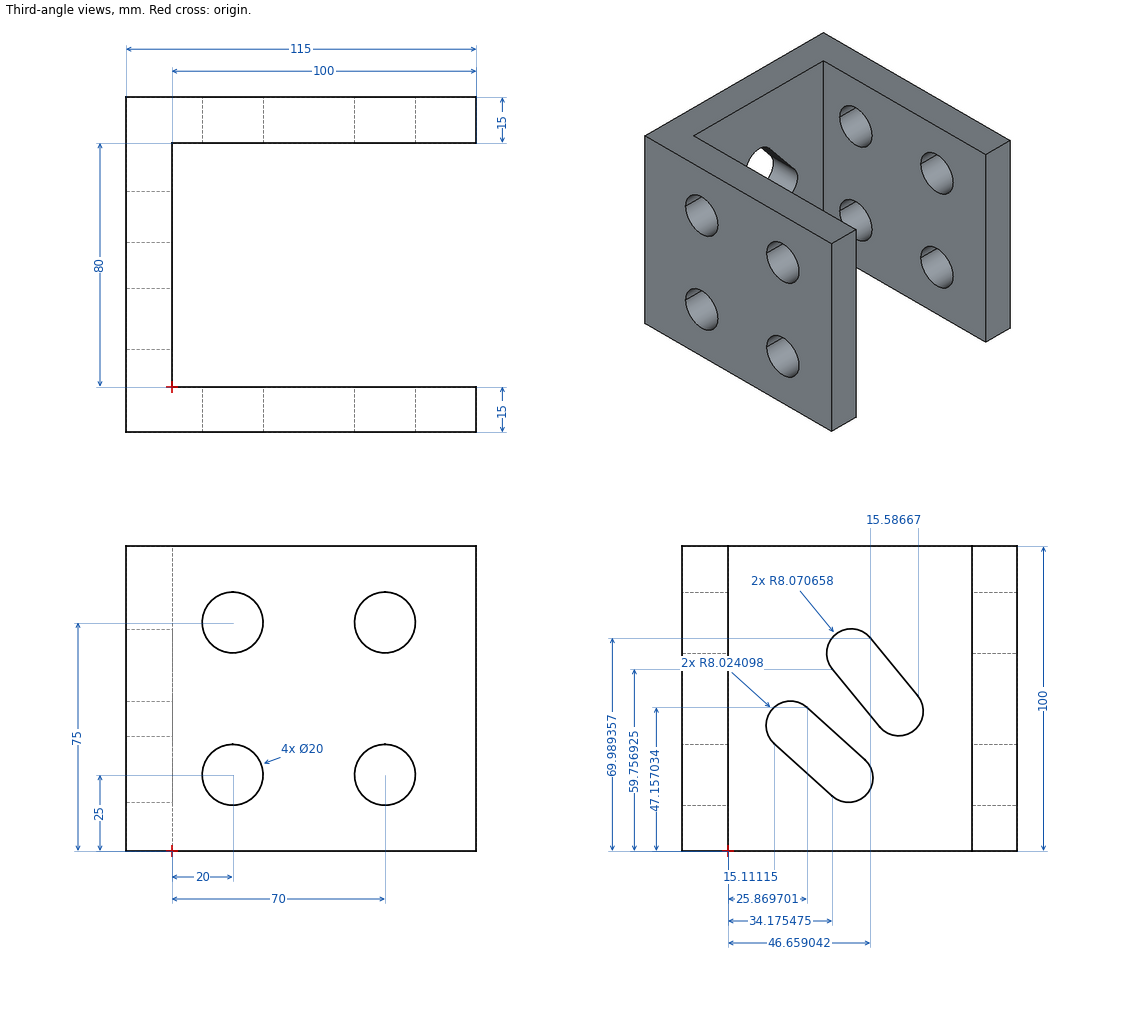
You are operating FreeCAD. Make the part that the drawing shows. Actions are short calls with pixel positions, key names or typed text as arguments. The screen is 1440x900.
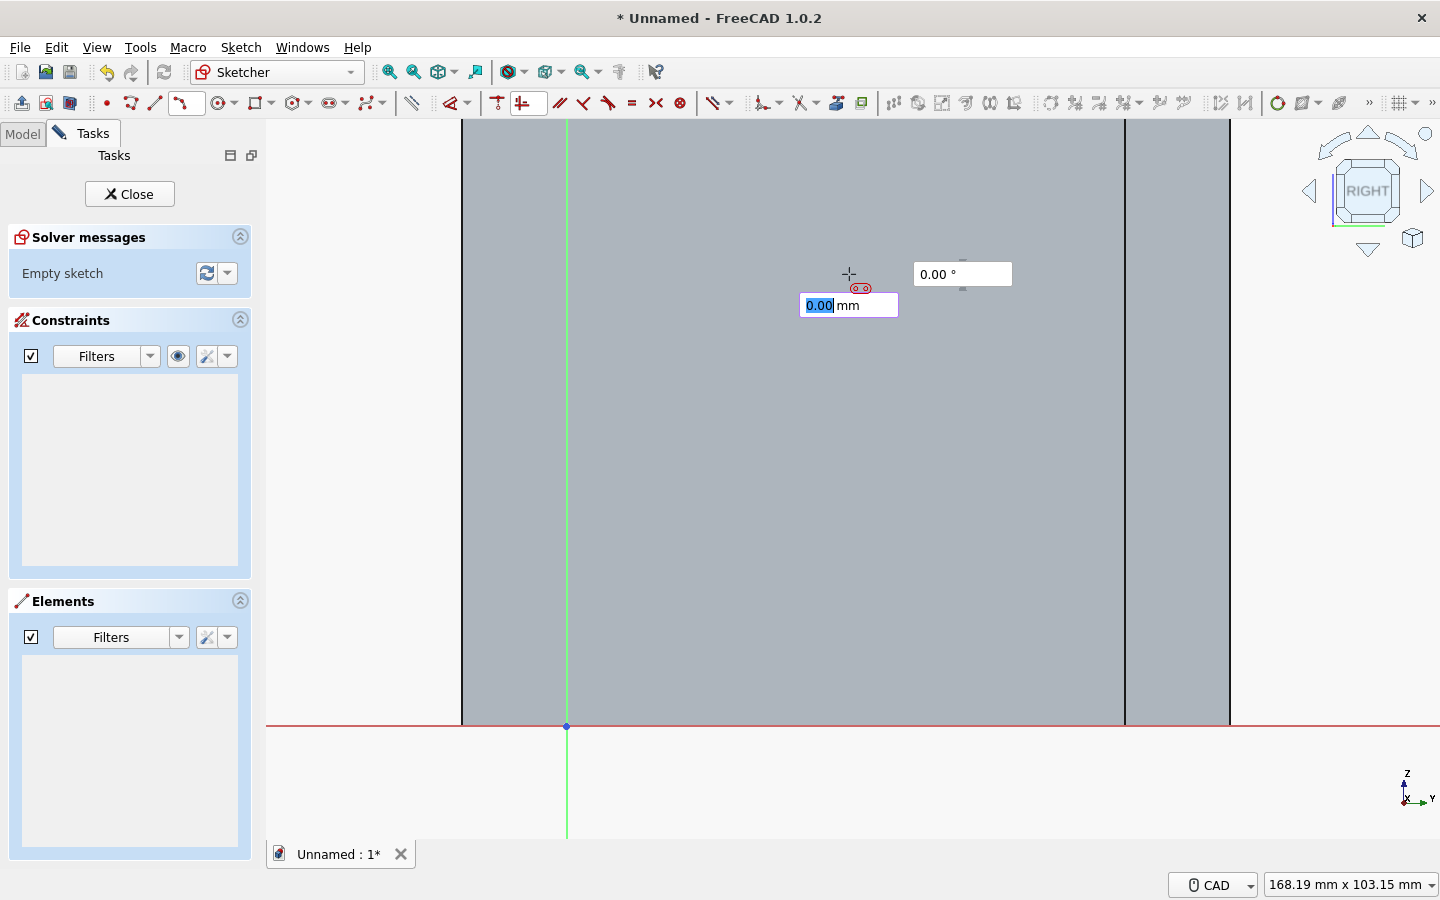
click(958, 406)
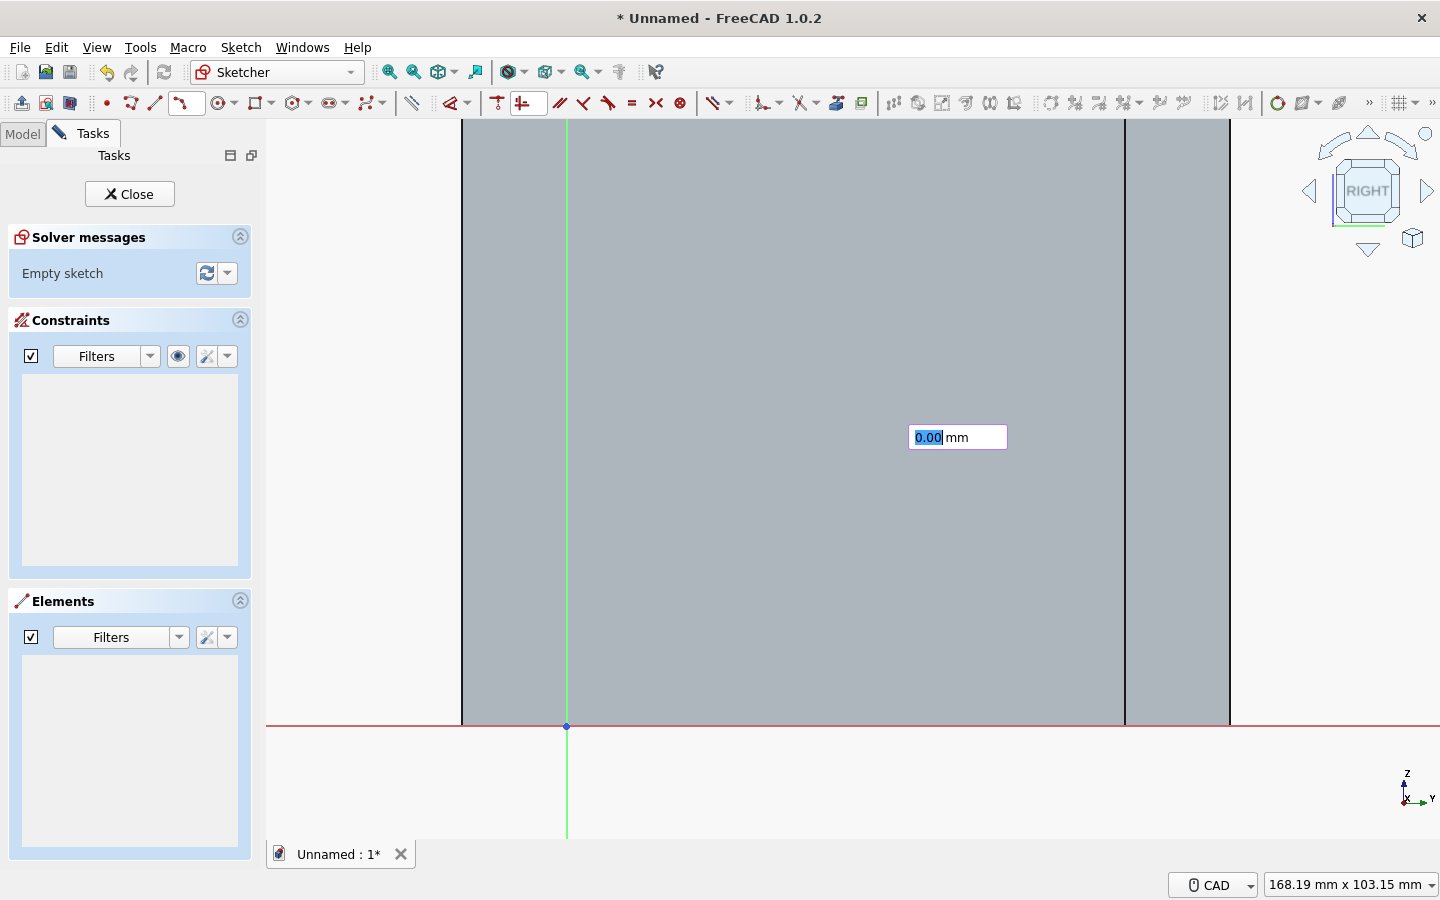
click(947, 304)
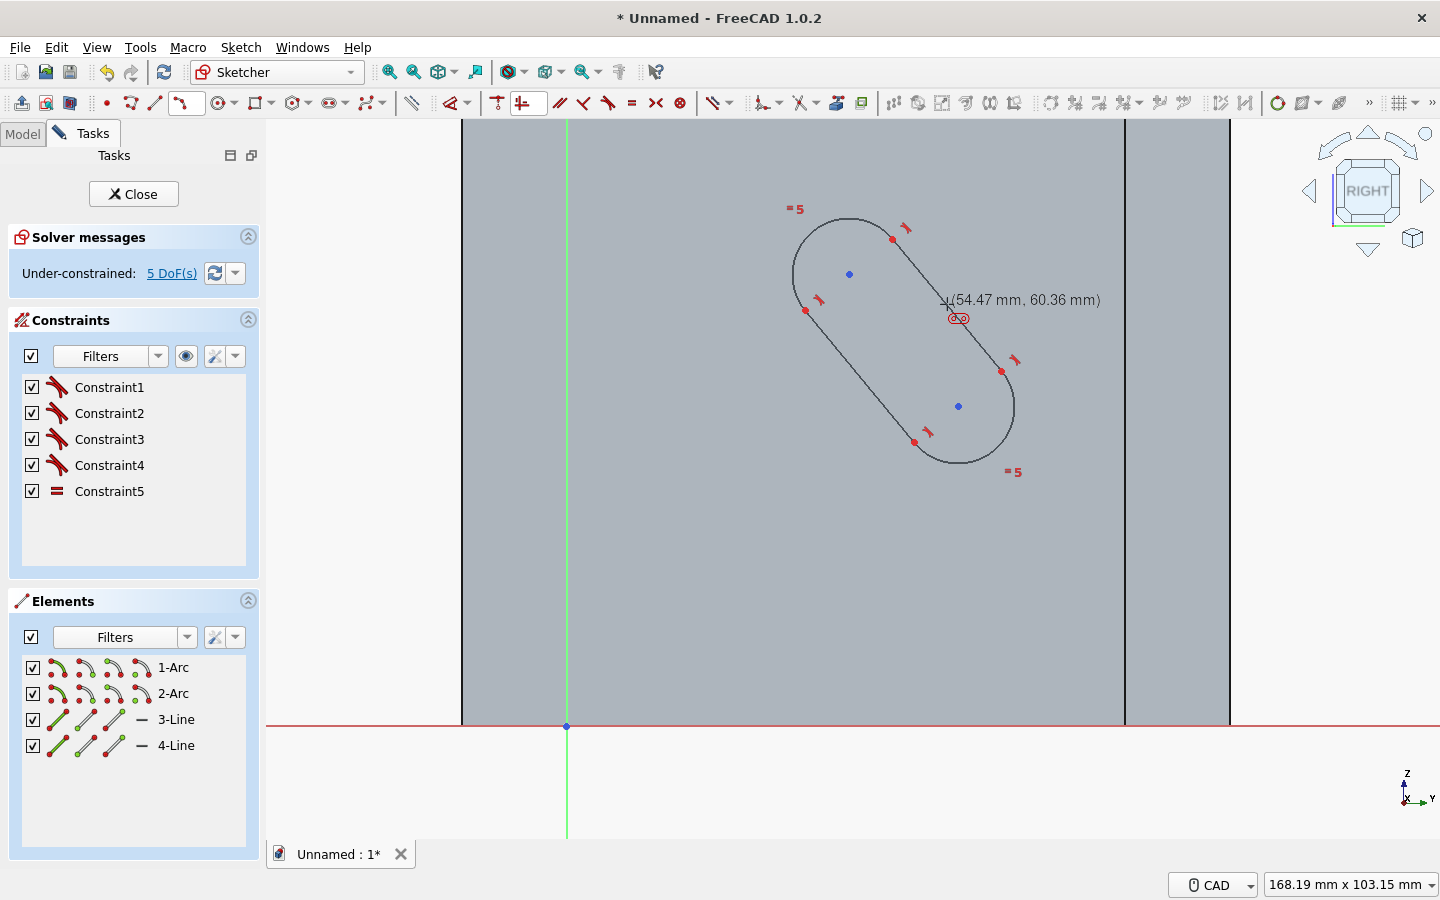
click(710, 439)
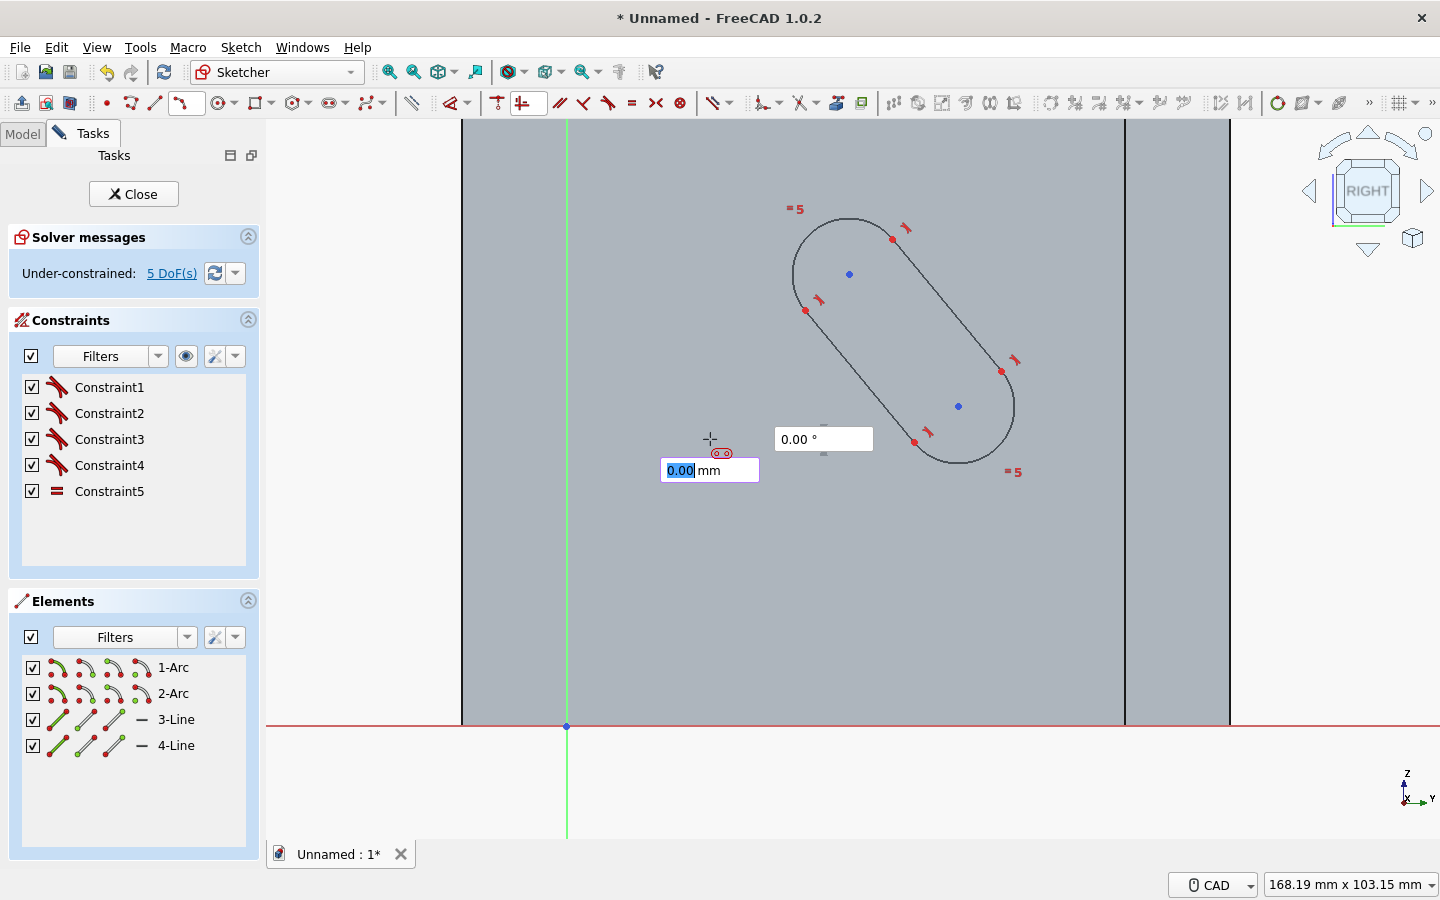
click(843, 559)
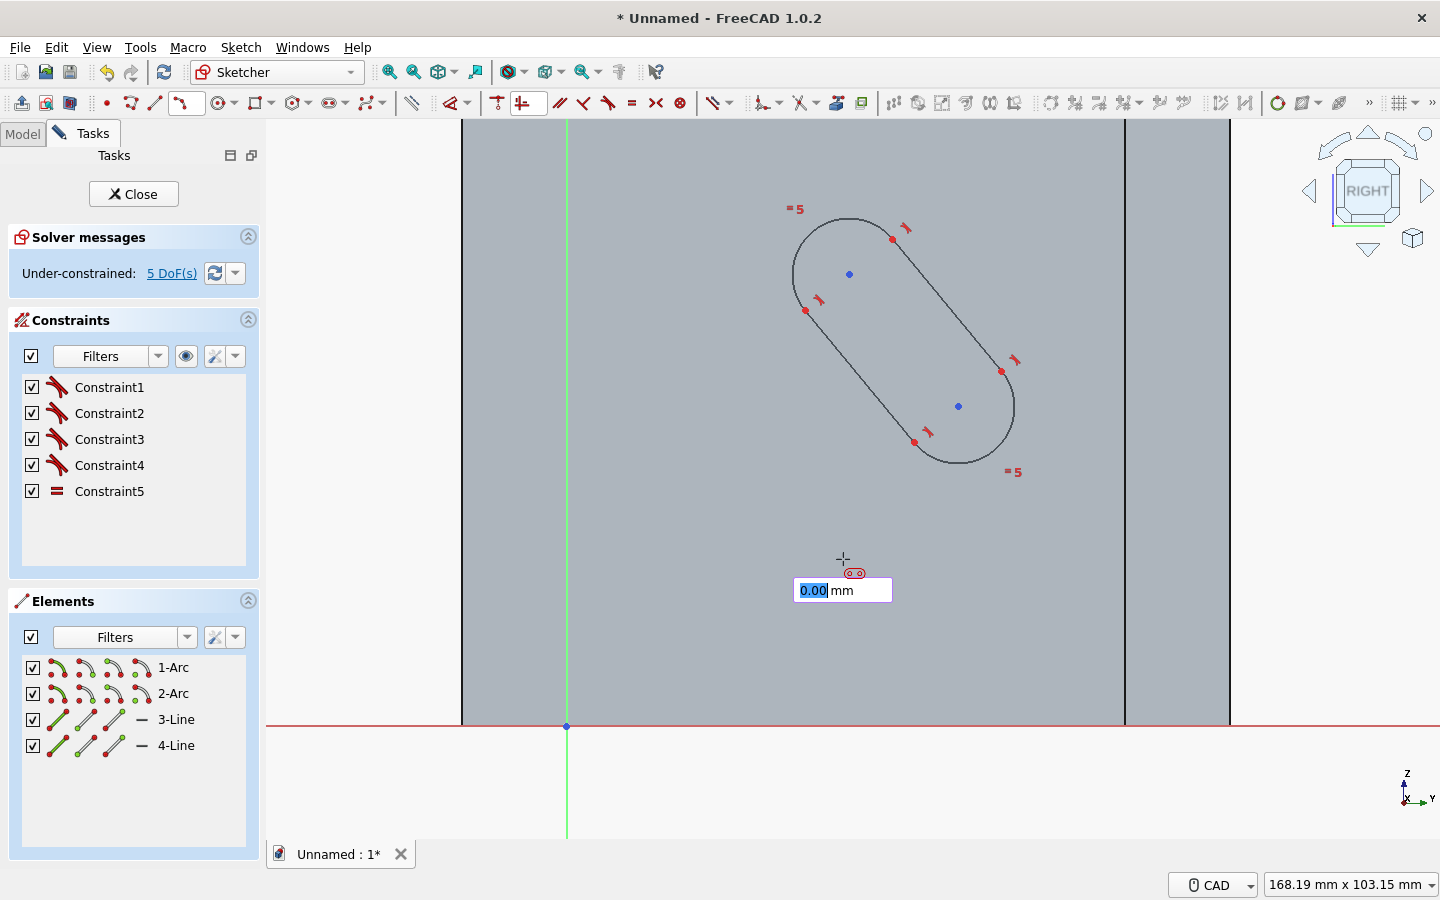
click(814, 457)
key(Escape)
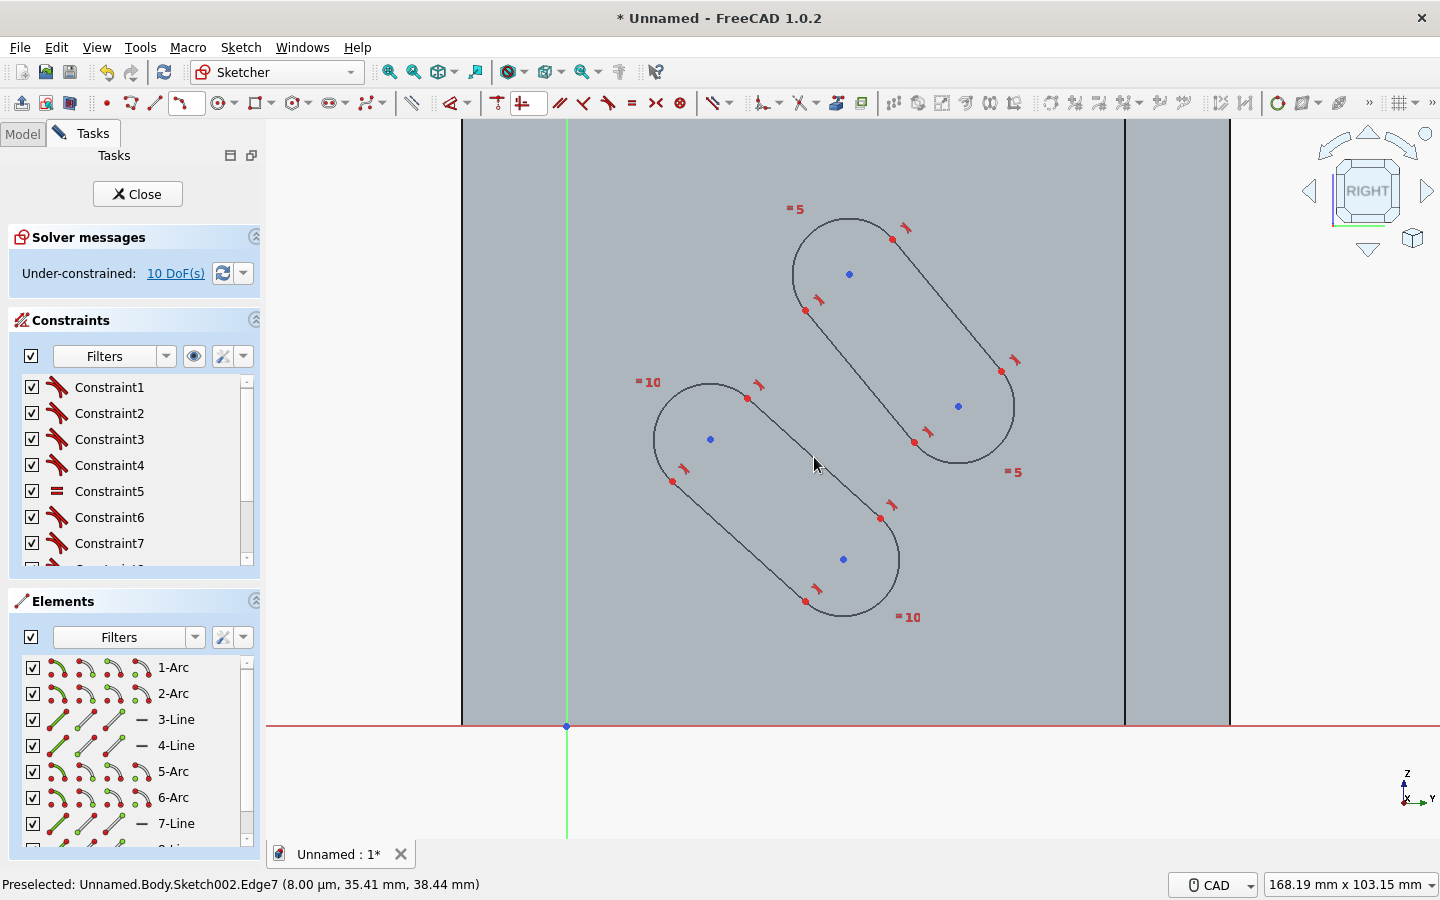
click(450, 104)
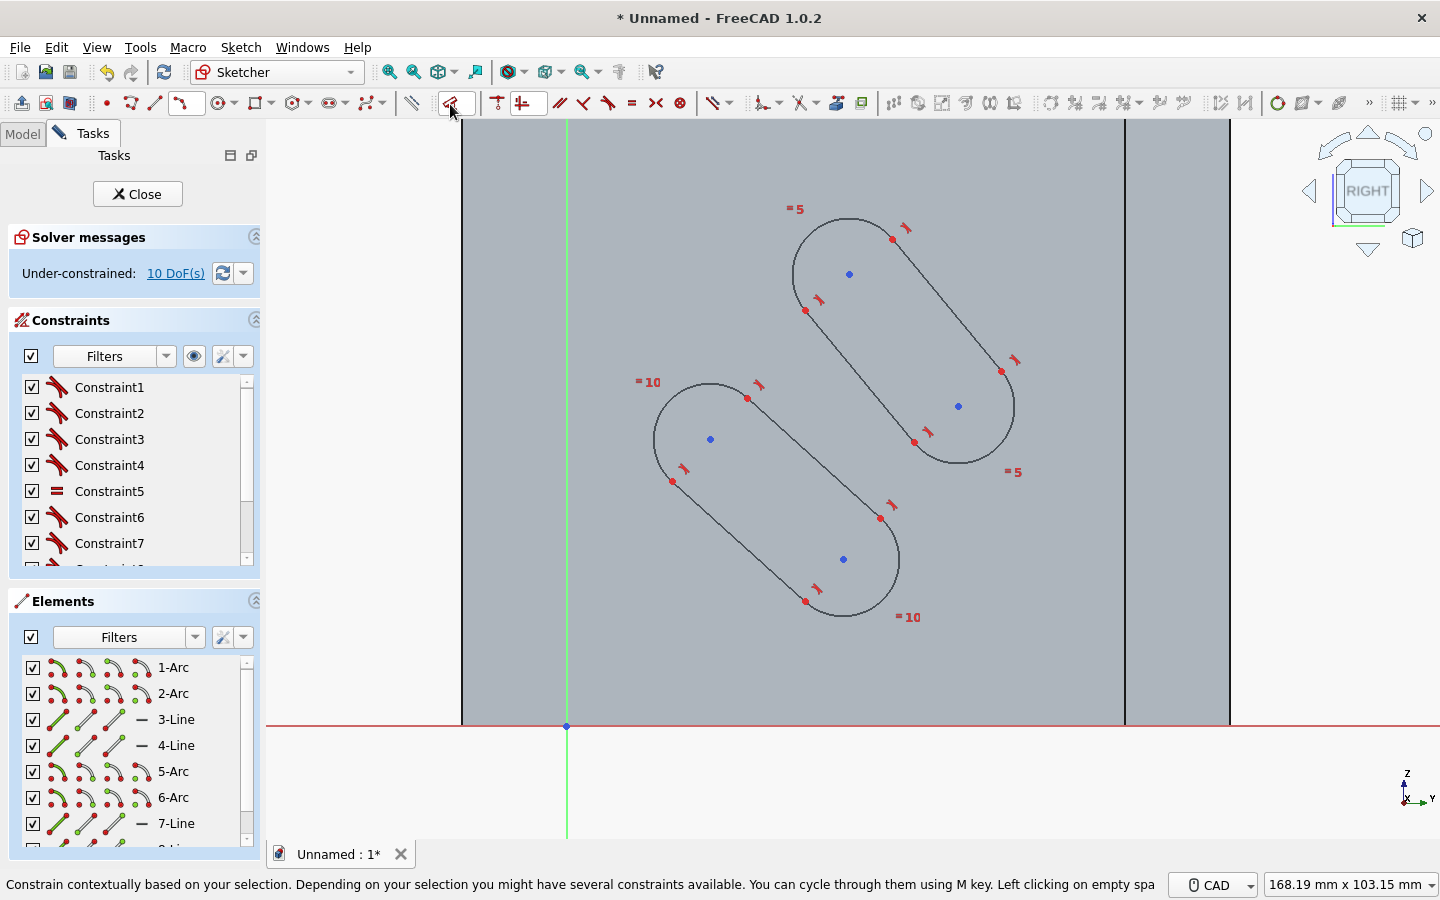
click(846, 219)
click(844, 187)